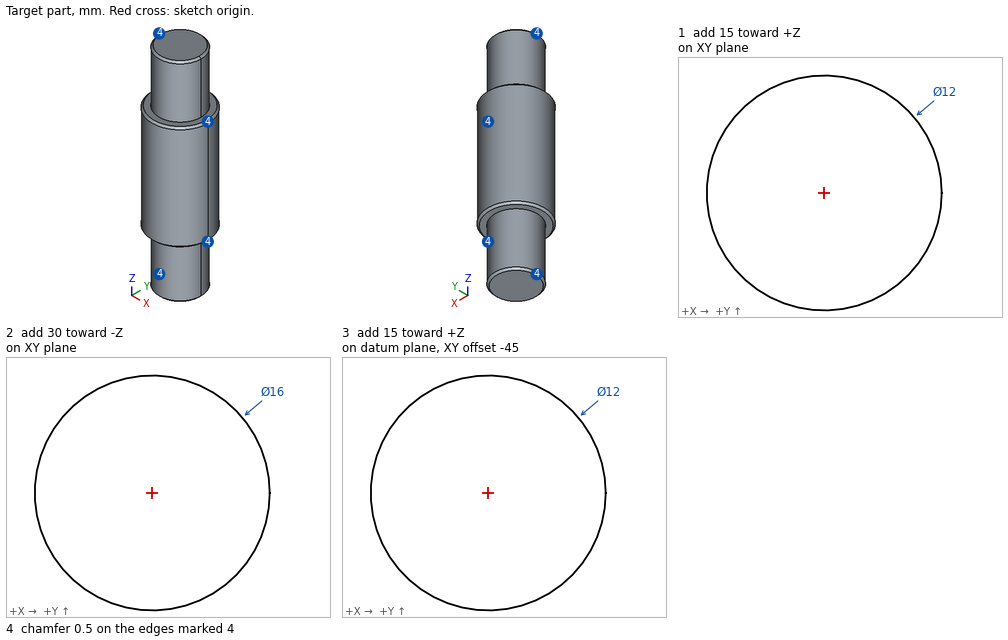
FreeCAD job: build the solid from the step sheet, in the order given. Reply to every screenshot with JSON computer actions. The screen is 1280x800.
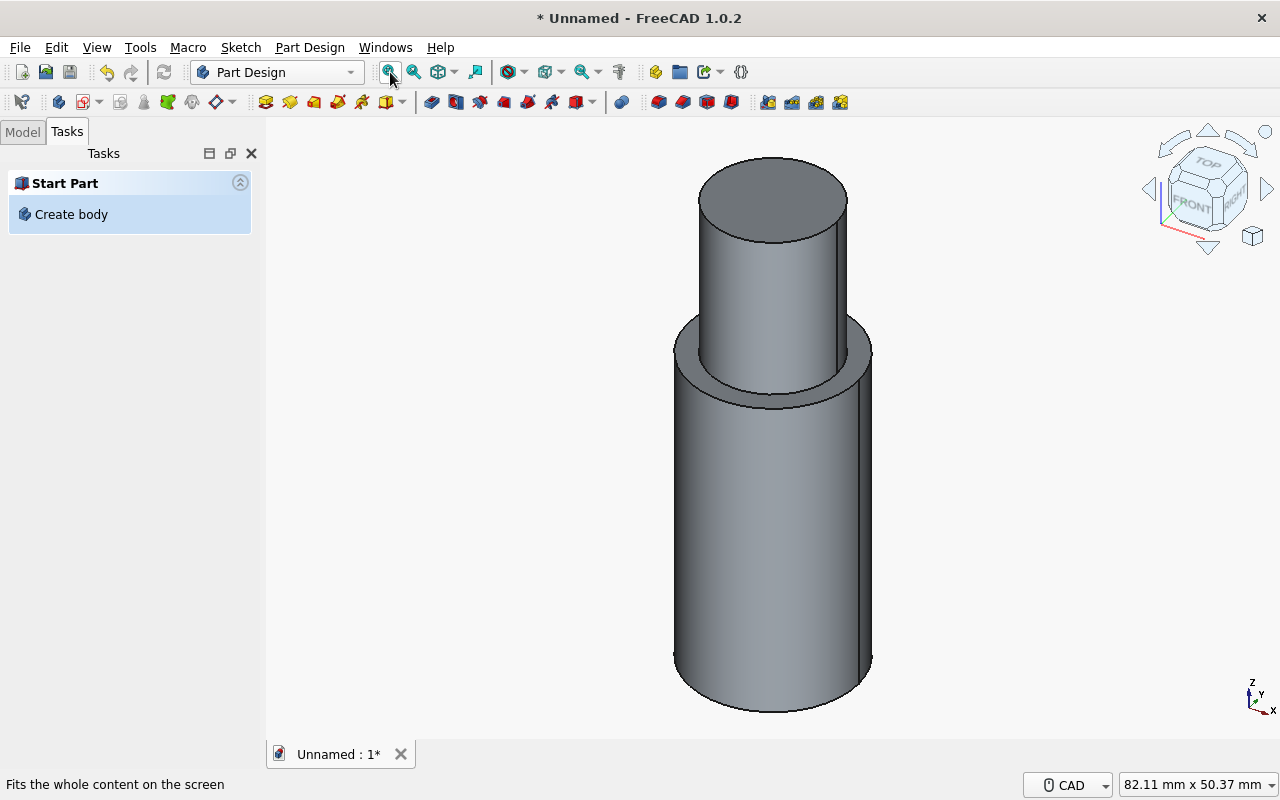
{"action": "left_click", "coordinate": [23, 131]}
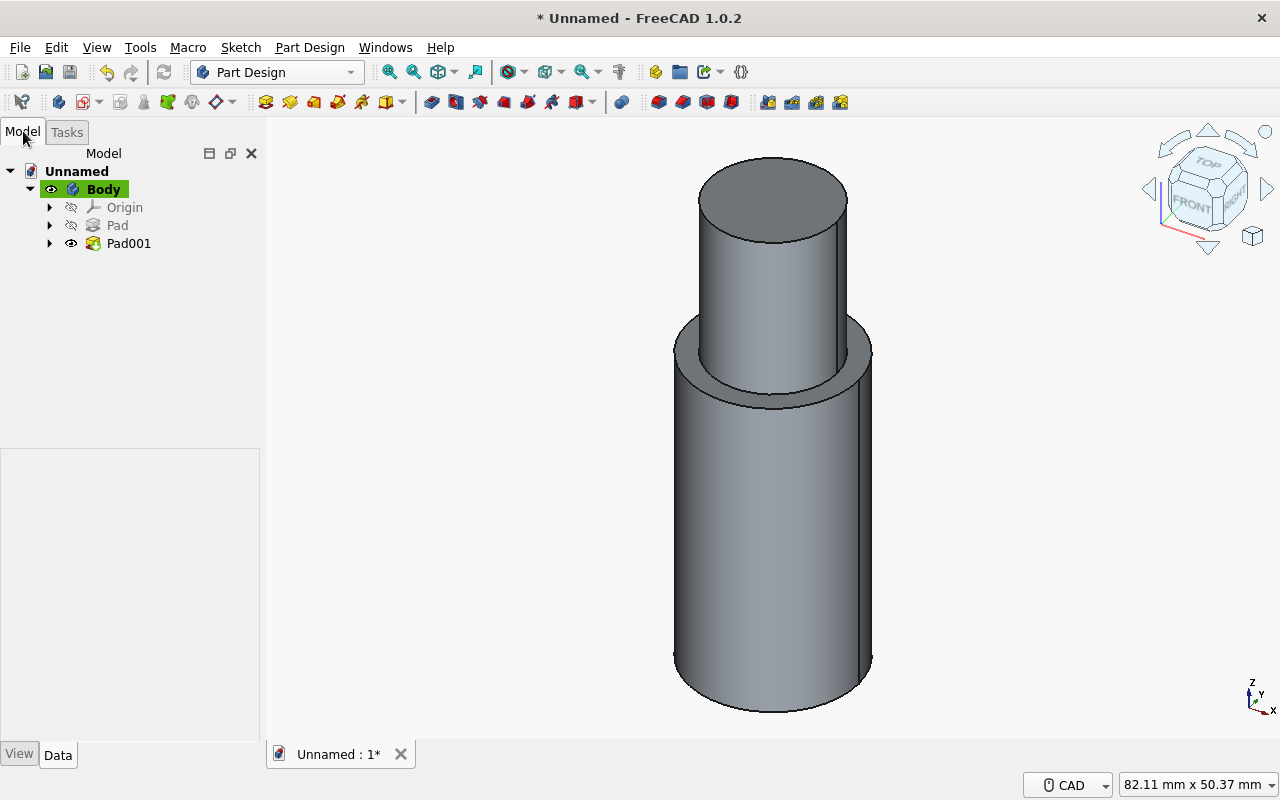
{"action": "left_click", "coordinate": [50, 207]}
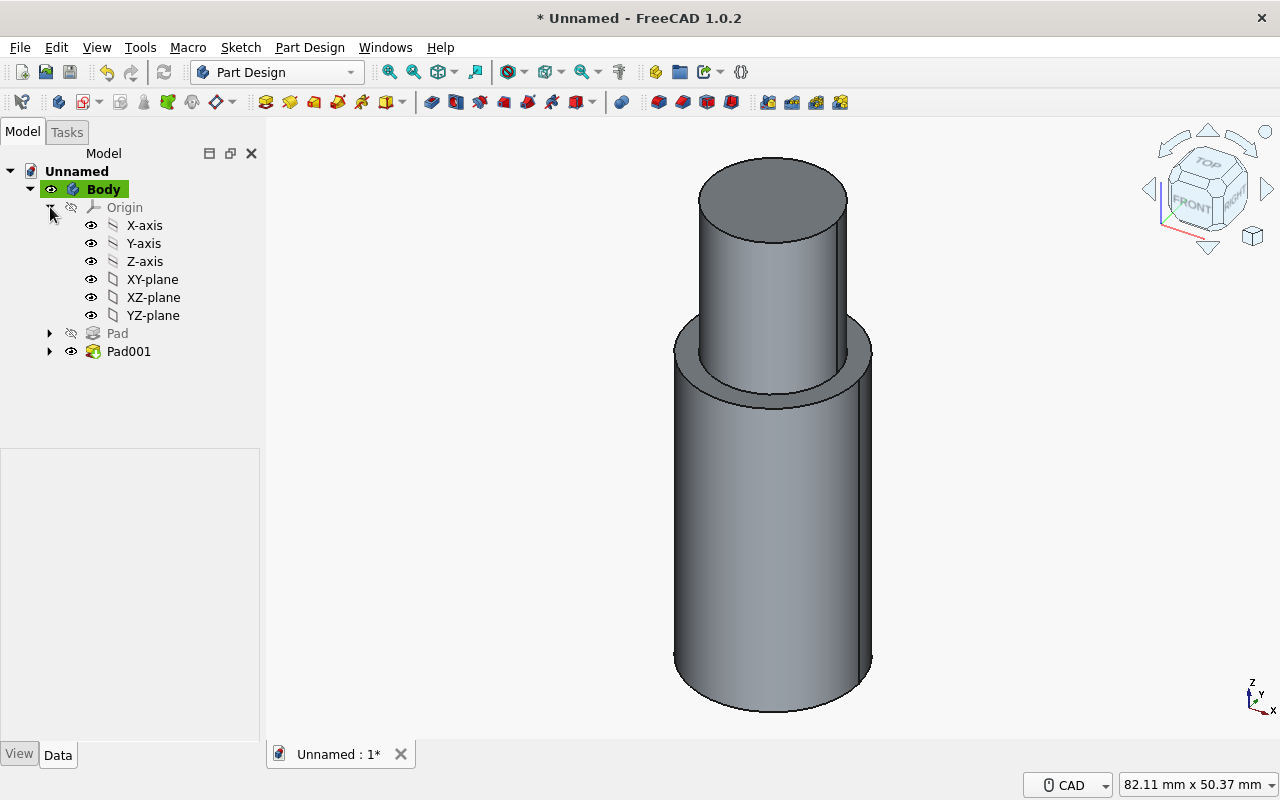
{"action": "left_click", "coordinate": [136, 279]}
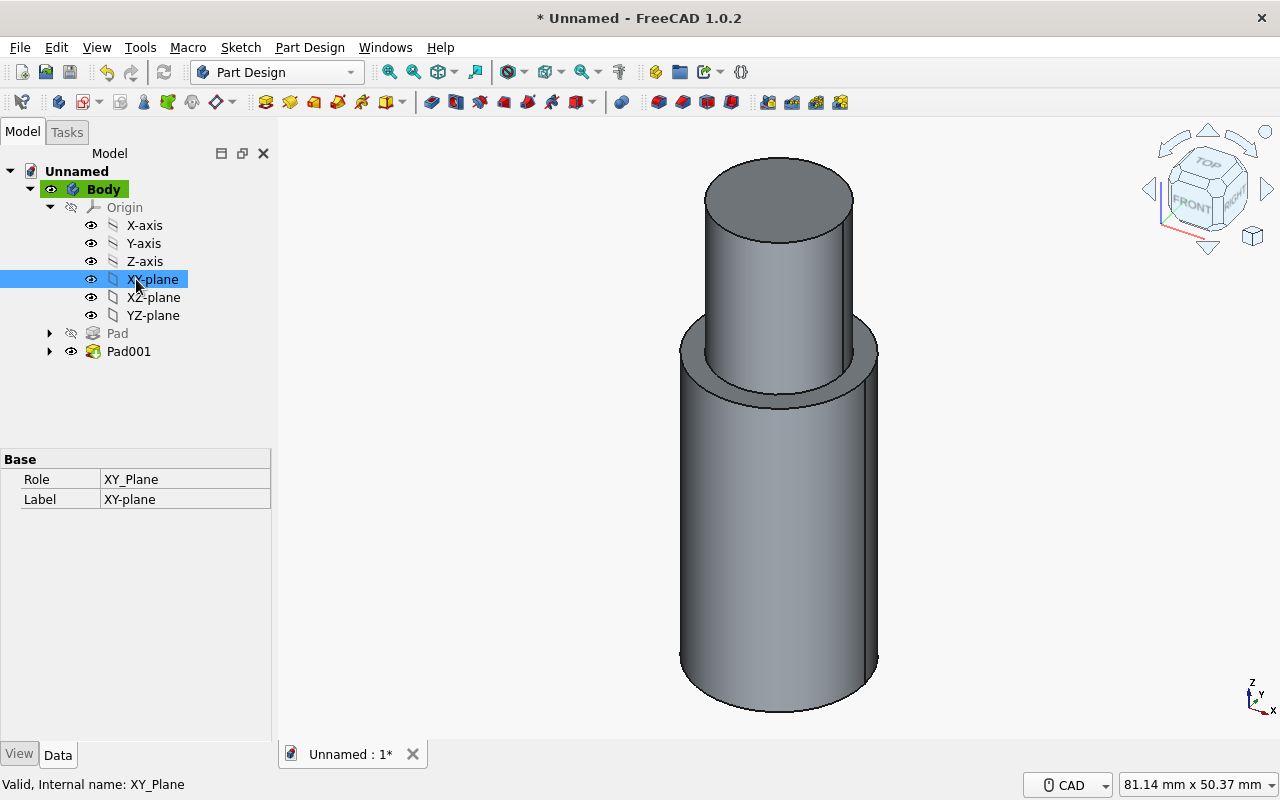
{"action": "left_click", "coordinate": [216, 102]}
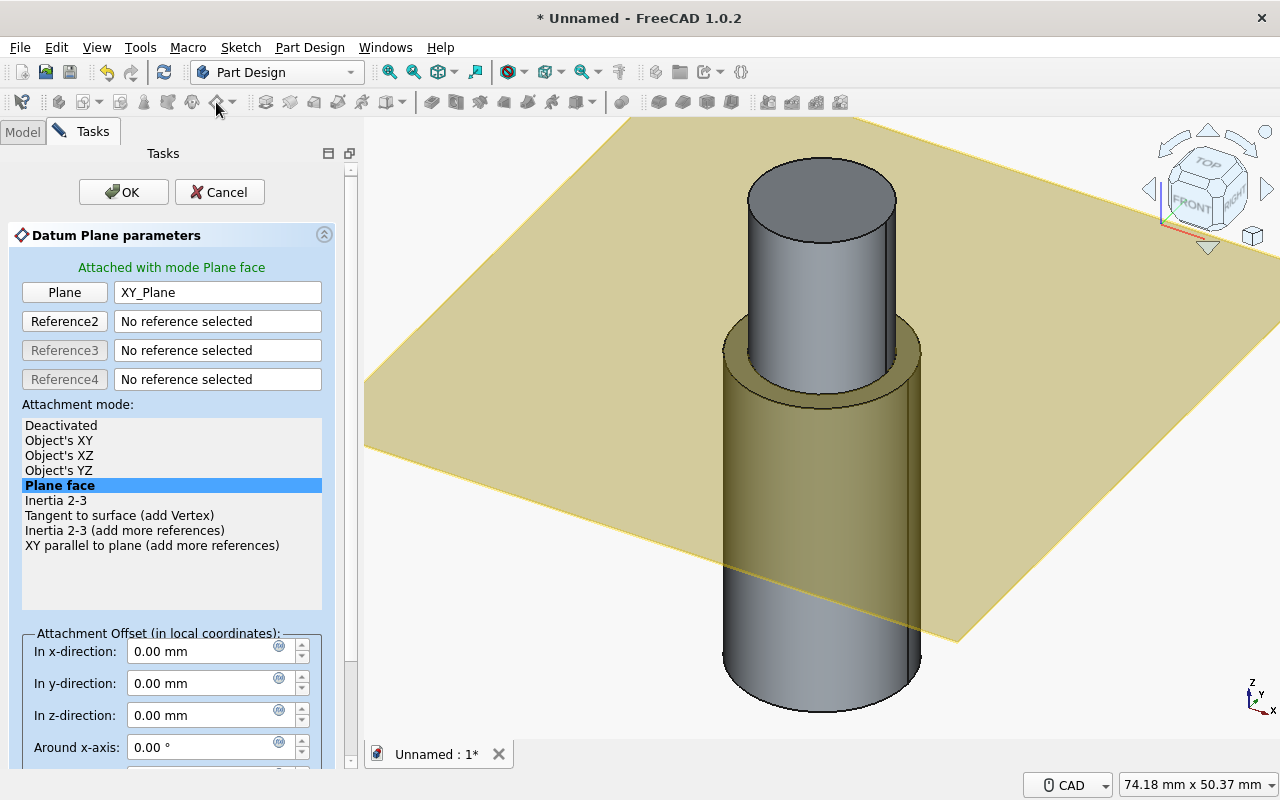
{"action": "triple_click", "coordinate": [210, 715]}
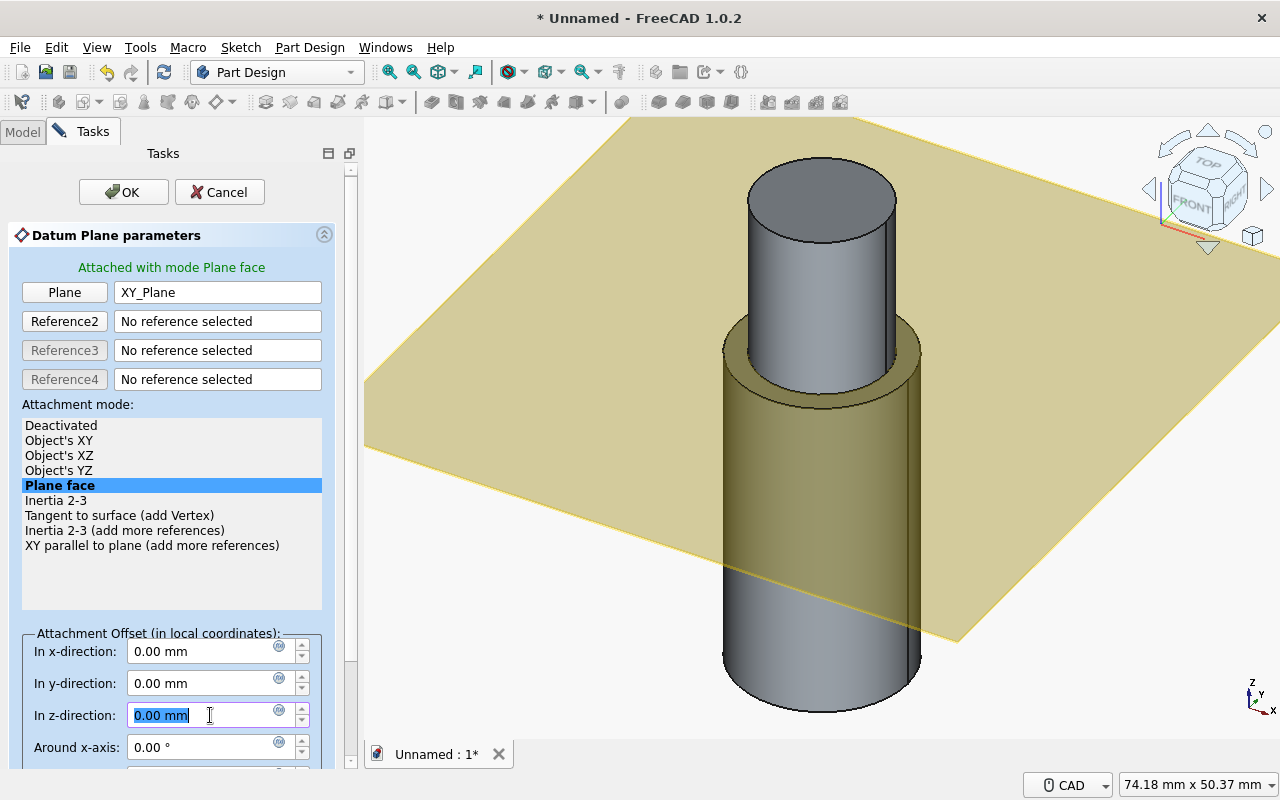
{"action": "type", "text": "-45"}
{"action": "key", "text": "Tab"}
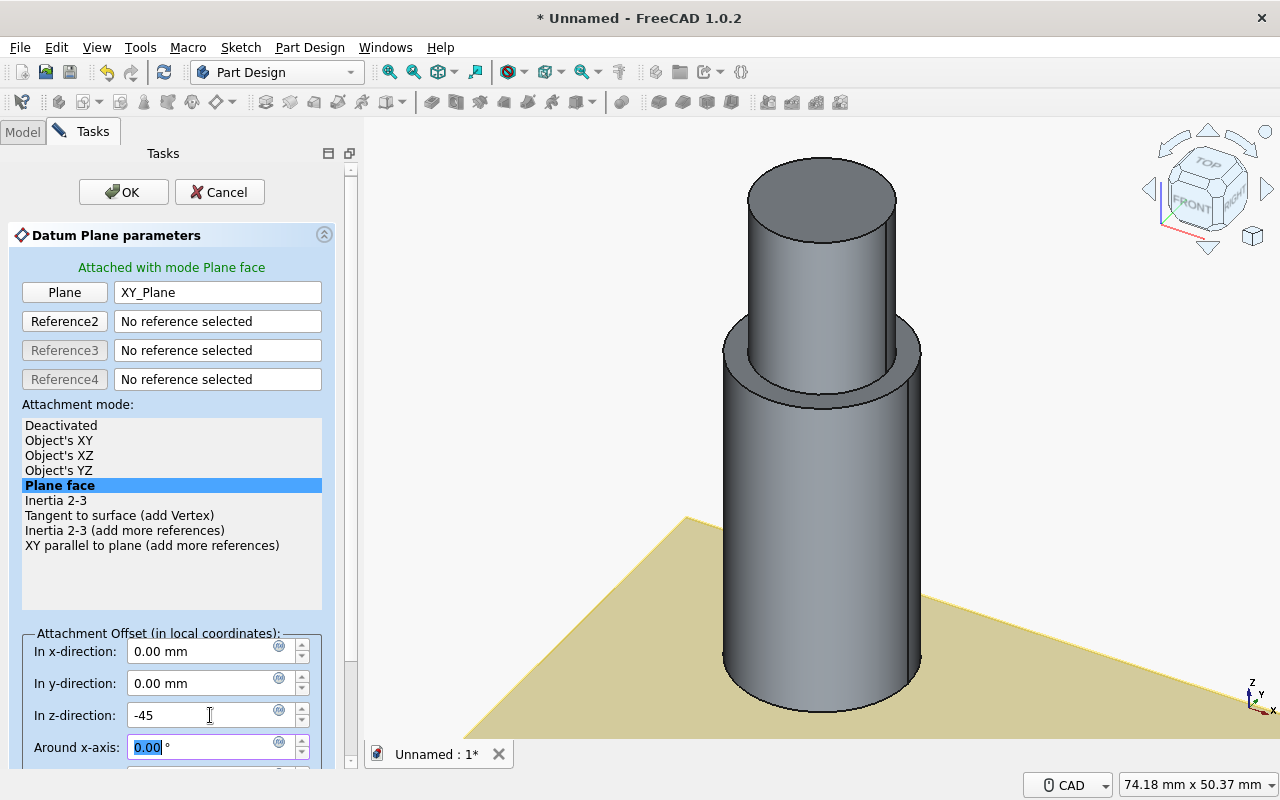
{"action": "left_click", "coordinate": [124, 192]}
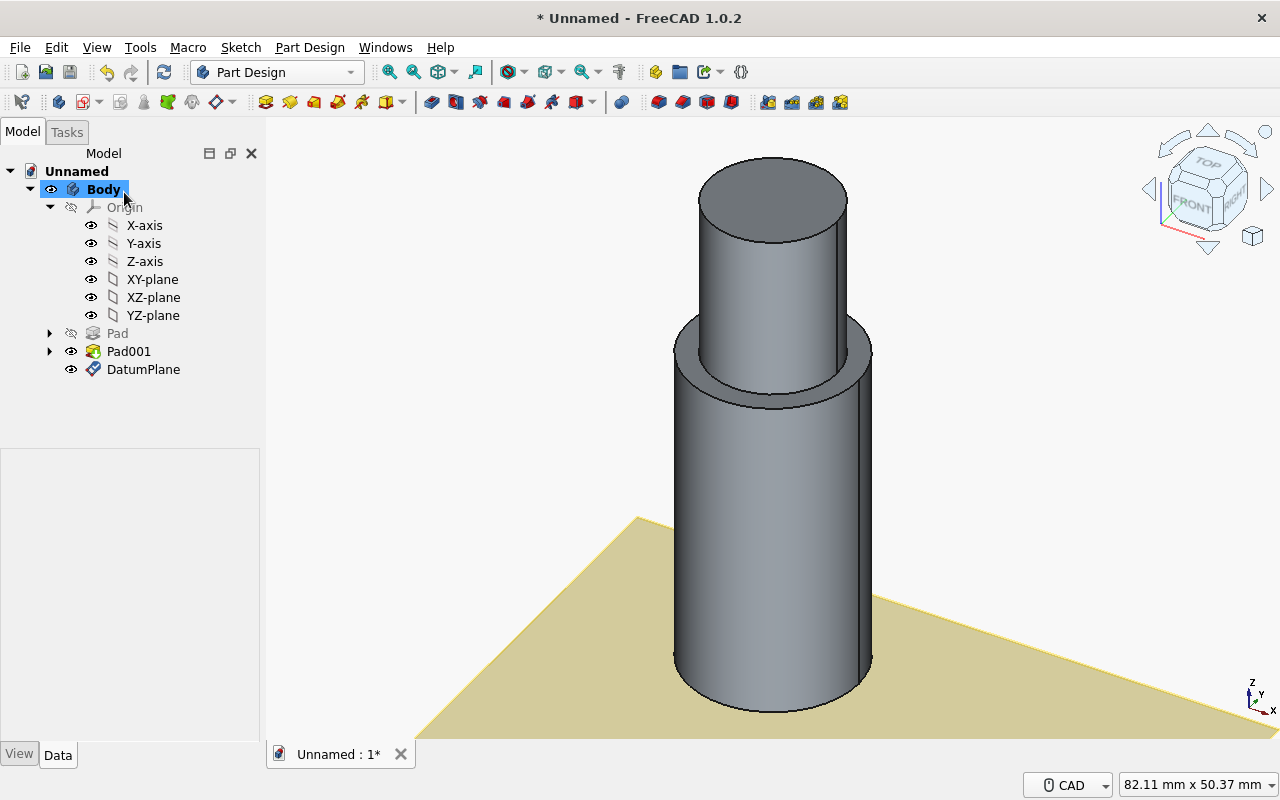
{"action": "left_click", "coordinate": [116, 369]}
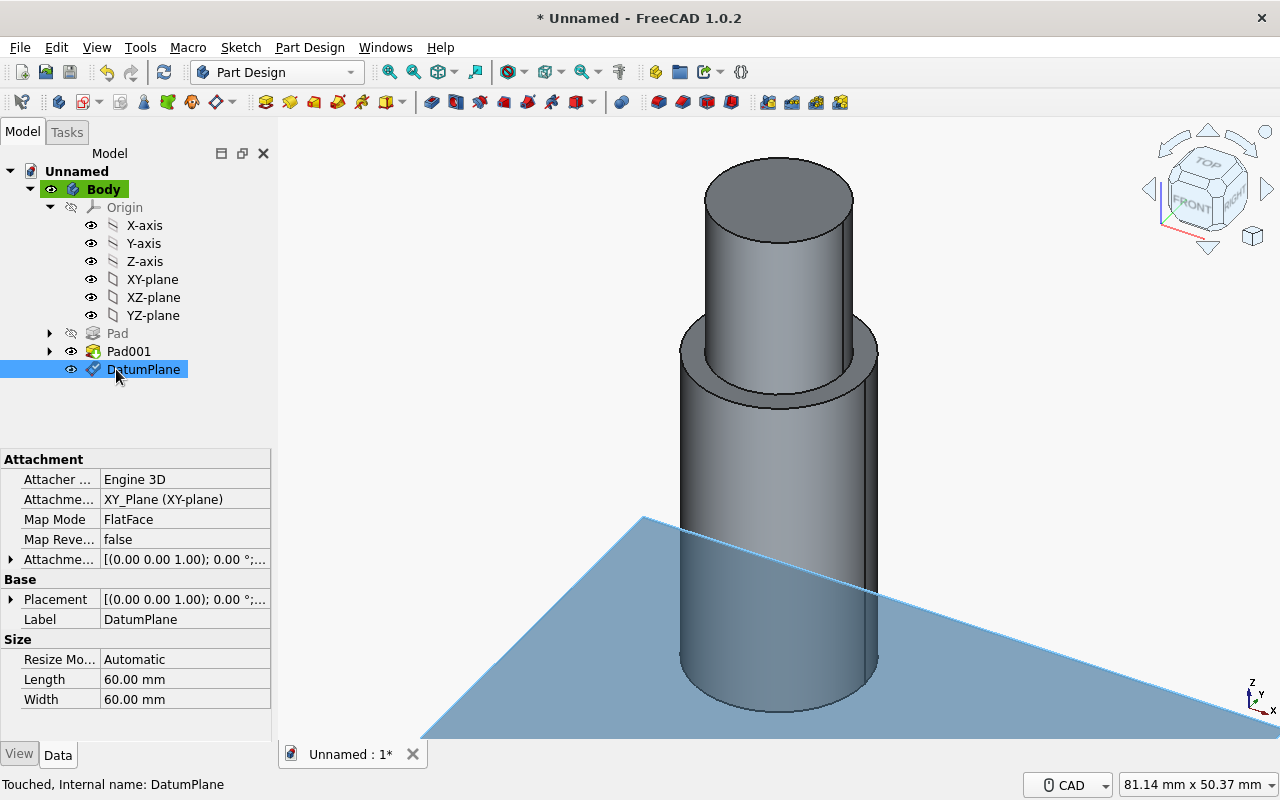
{"action": "left_click", "coordinate": [84, 102]}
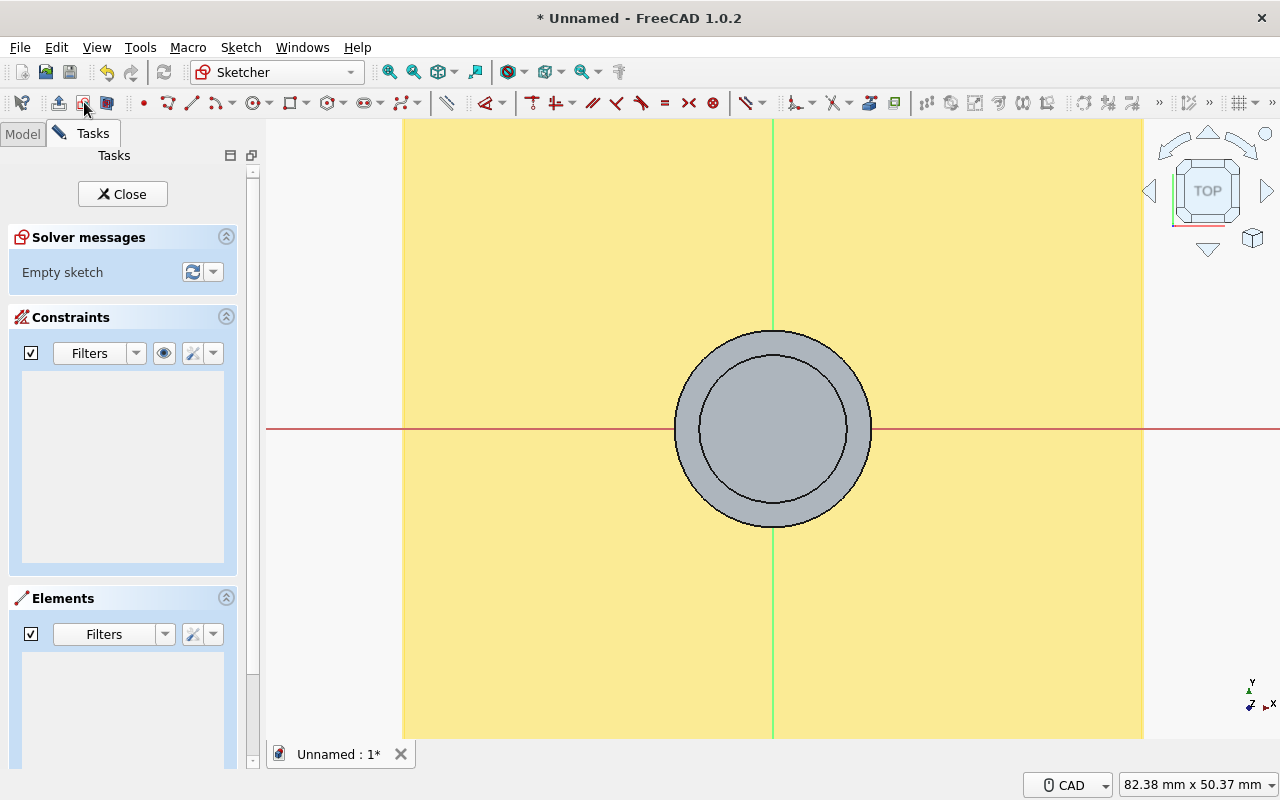
{"action": "left_click", "coordinate": [108, 104]}